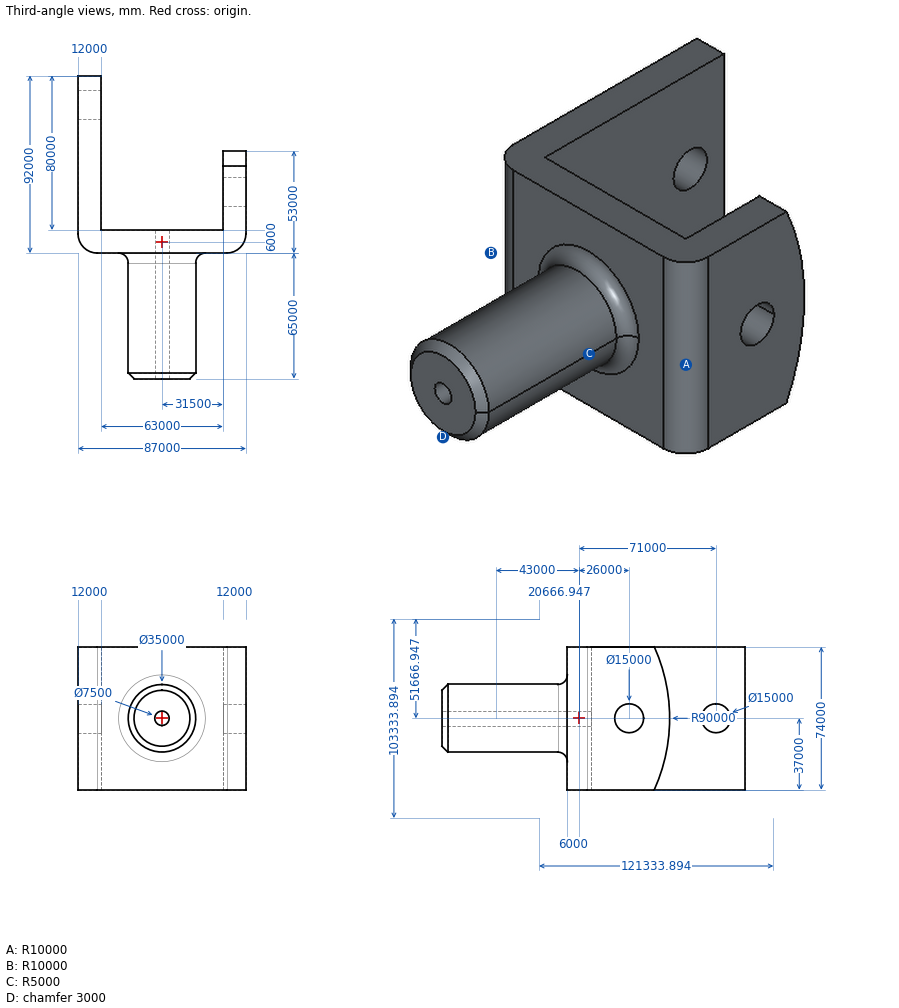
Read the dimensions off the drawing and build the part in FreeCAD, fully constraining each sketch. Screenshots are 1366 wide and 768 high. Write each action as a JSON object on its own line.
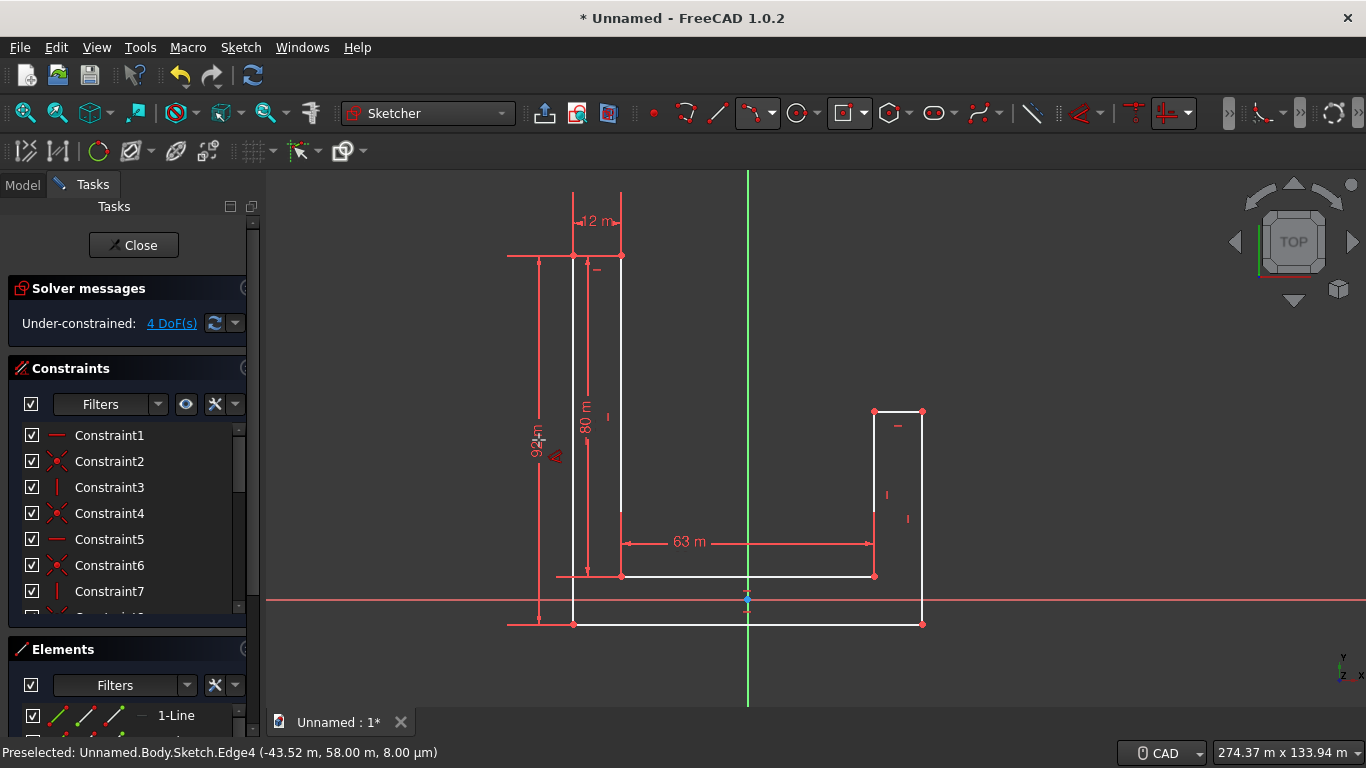
{"action": "left_click", "coordinate": [678, 625]}
{"action": "left_click", "coordinate": [667, 659]}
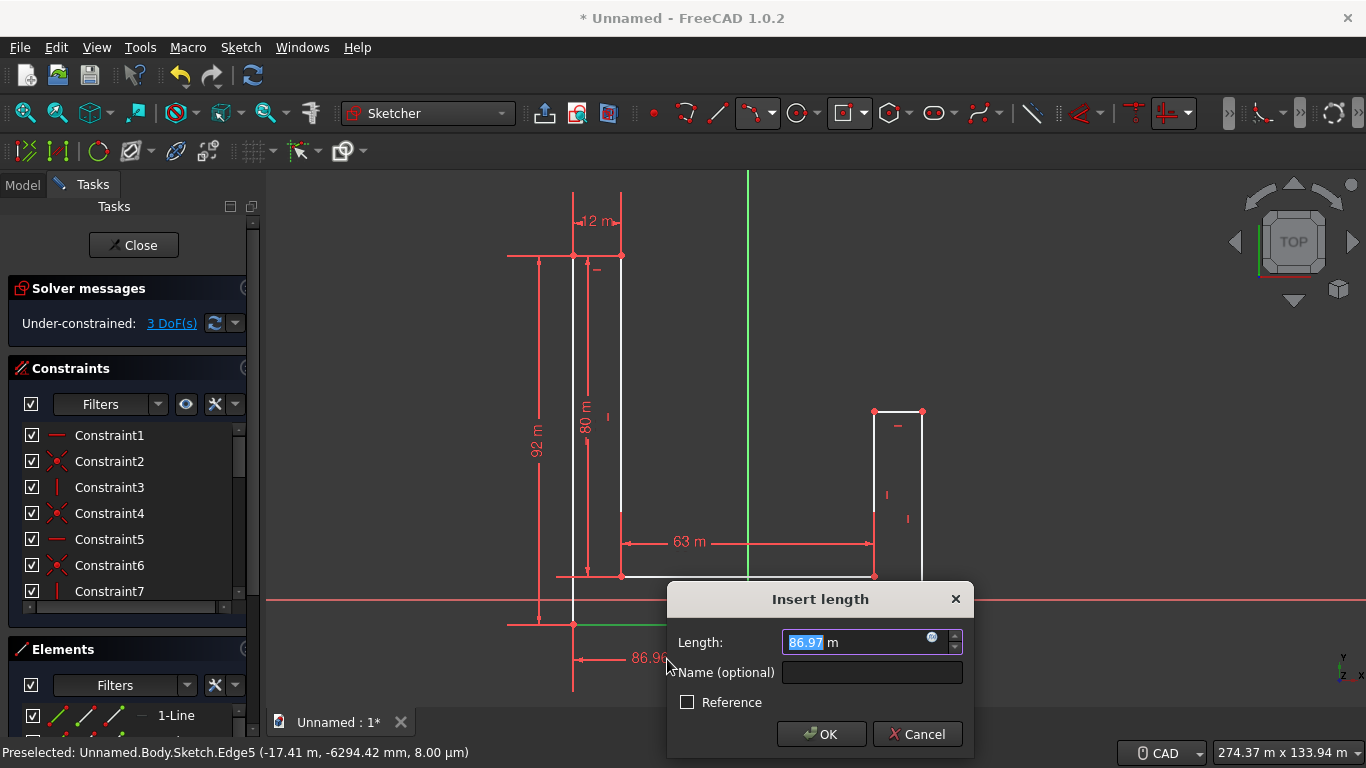
{"action": "key", "text": "ctrl+a"}
{"action": "type", "text": "87000 mm"}
{"action": "key", "text": "Return"}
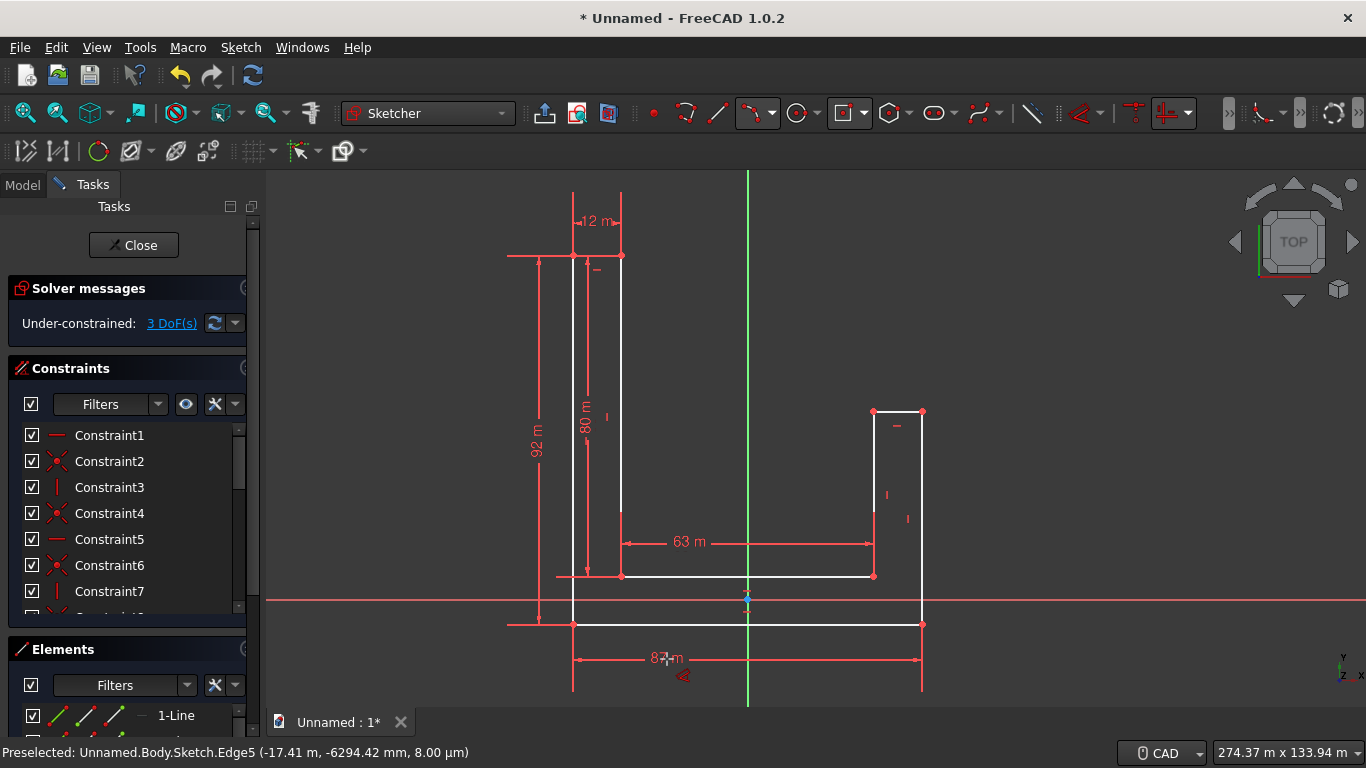
{"action": "left_click", "coordinate": [922, 561]}
{"action": "left_click", "coordinate": [956, 518]}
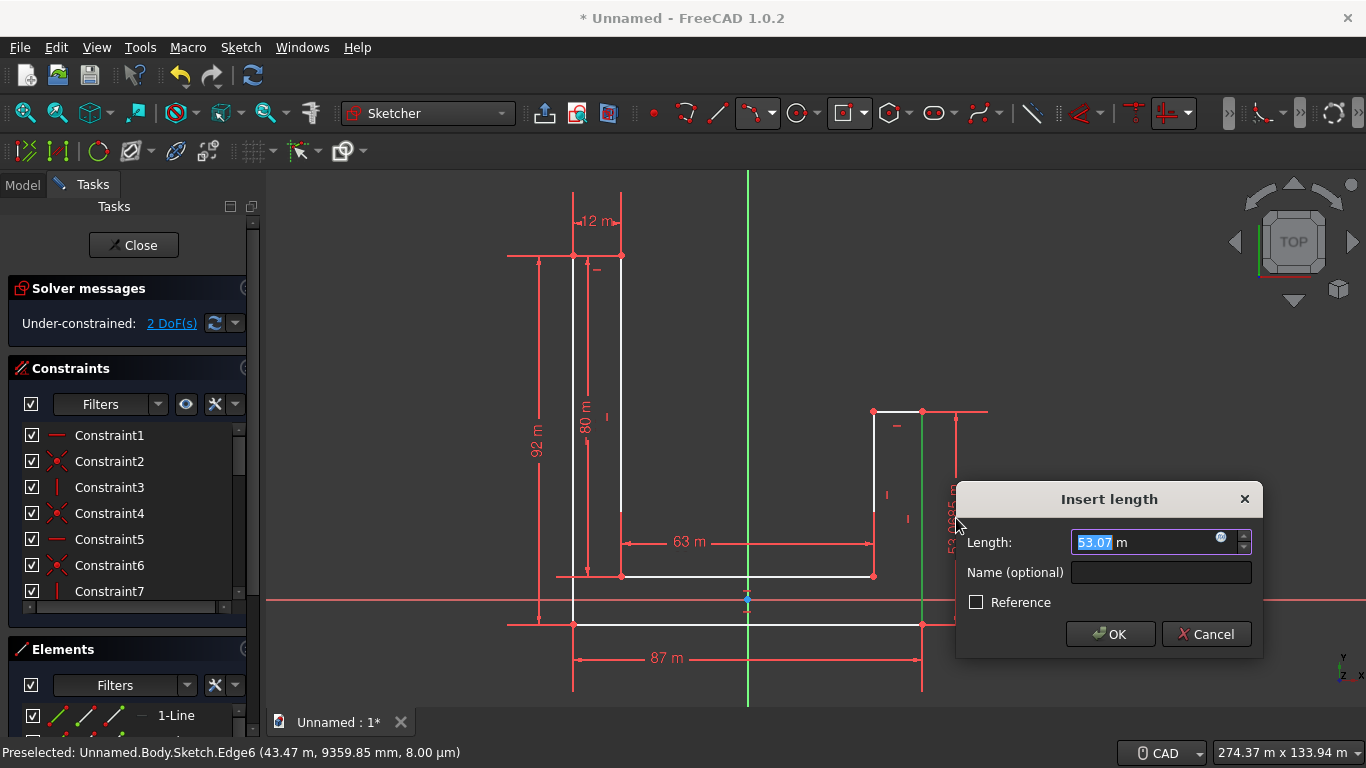
{"action": "key", "text": "ctrl+a"}
{"action": "type", "text": "53000 mm"}
{"action": "key", "text": "Return"}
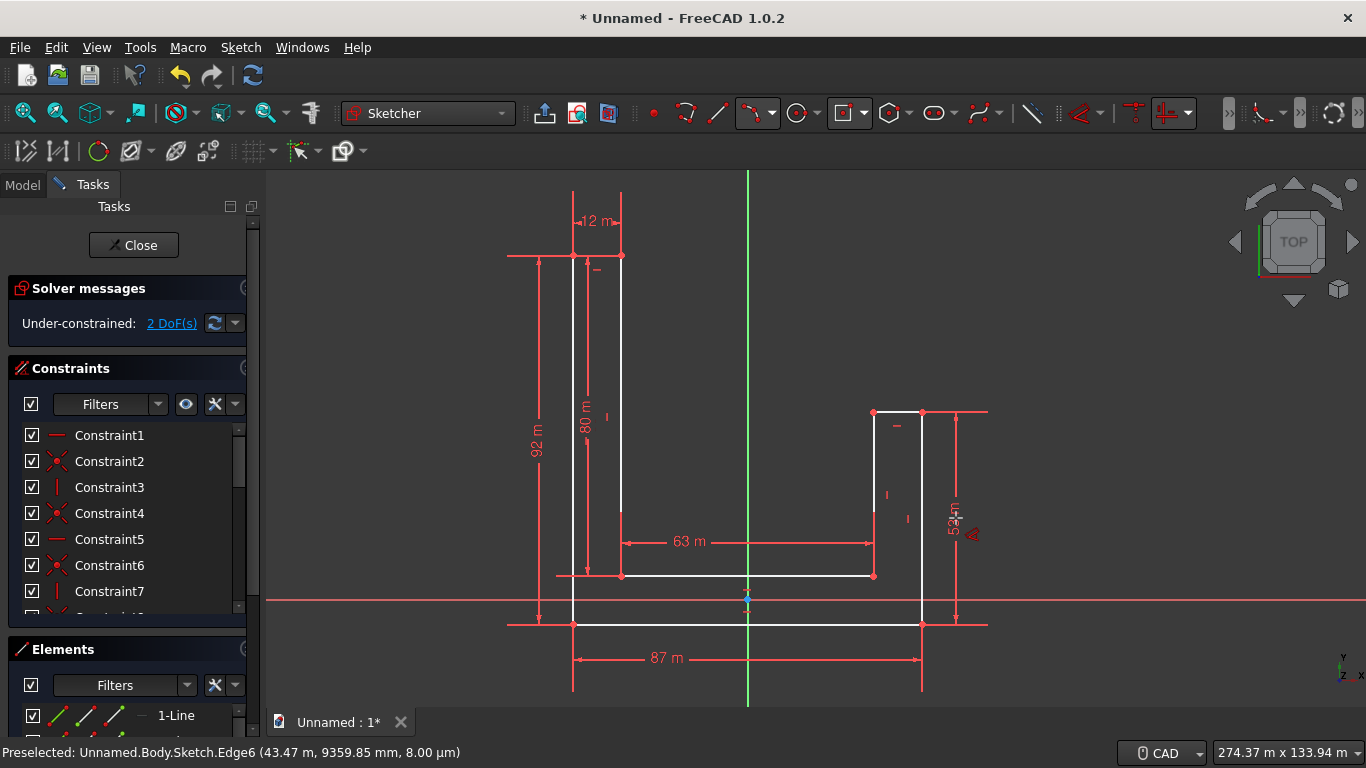
{"action": "scroll", "coordinate": [874, 576], "scroll_direction": "up", "scroll_amount": 3}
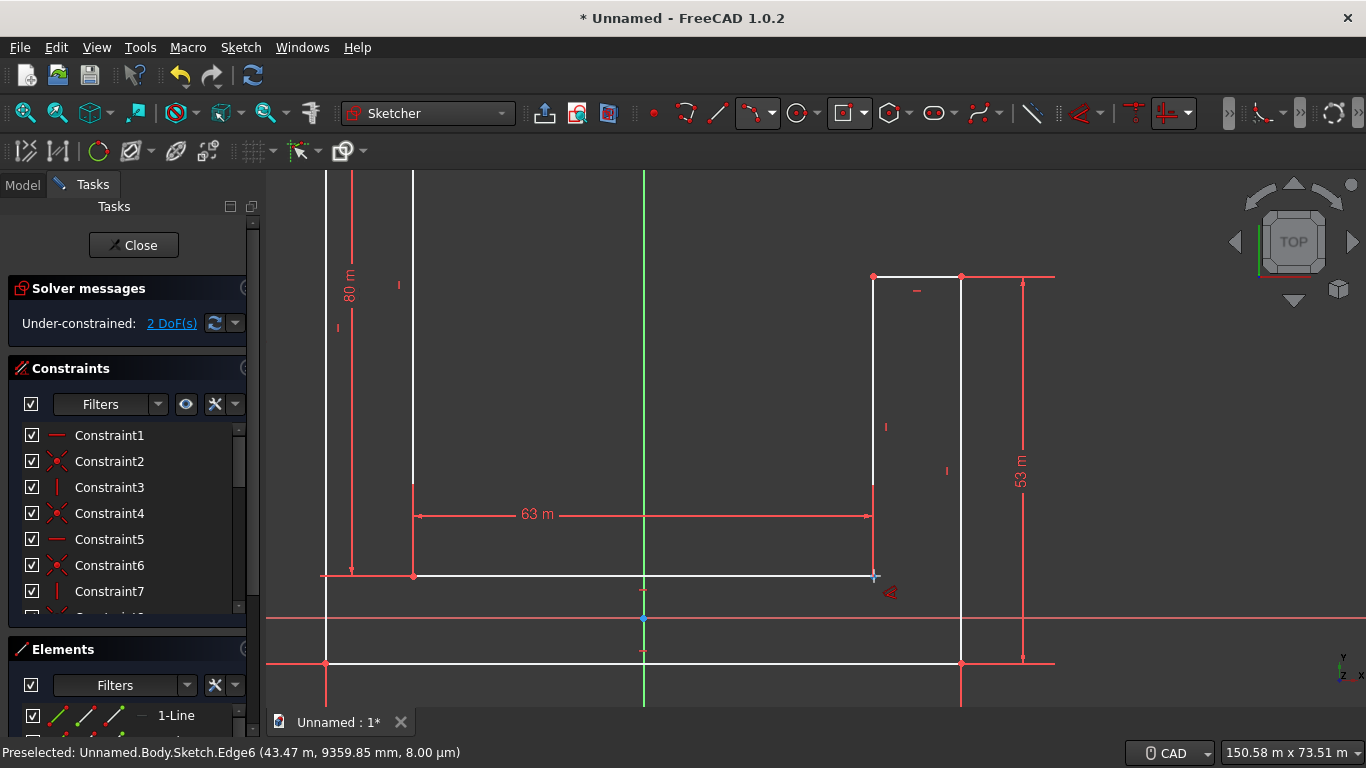
{"action": "left_click", "coordinate": [873, 576]}
{"action": "left_click", "coordinate": [907, 597]}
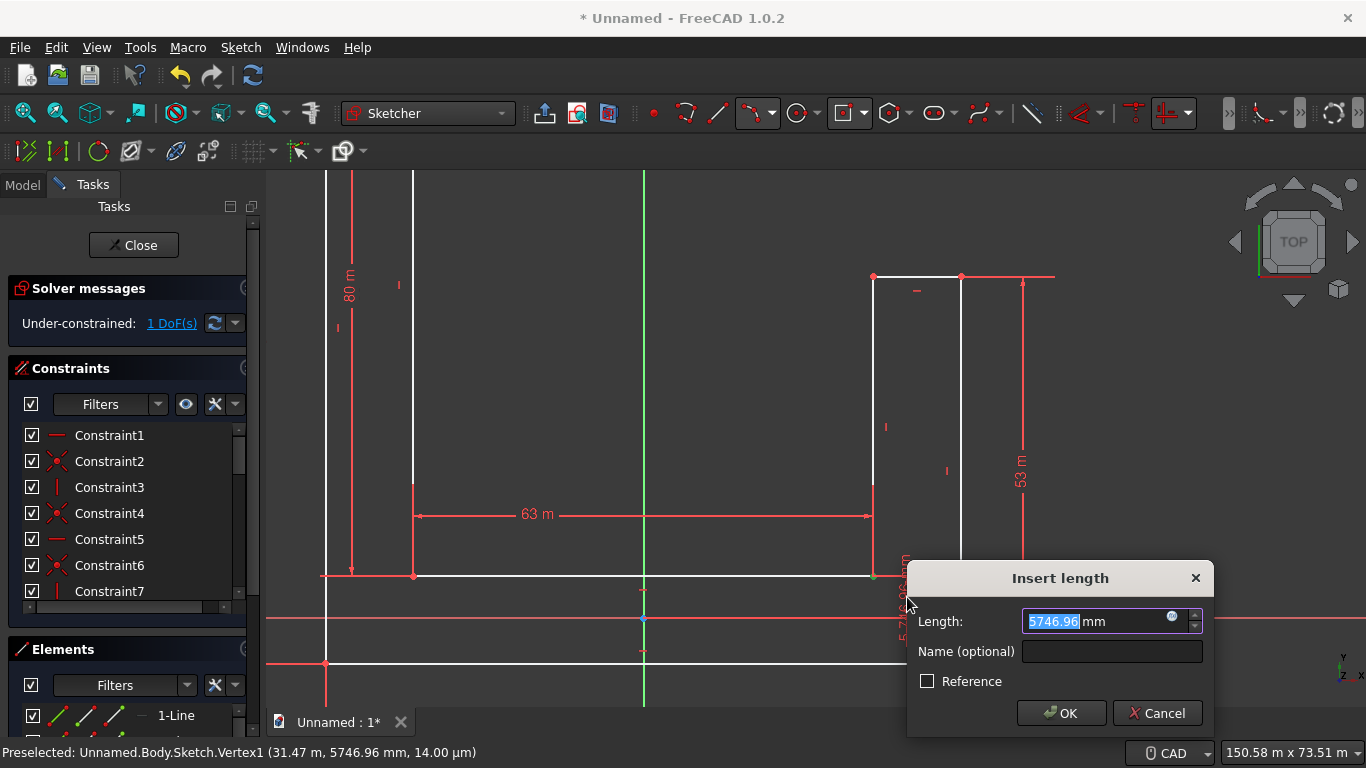
{"action": "type", "text": "6000"}
{"action": "key", "text": "Return"}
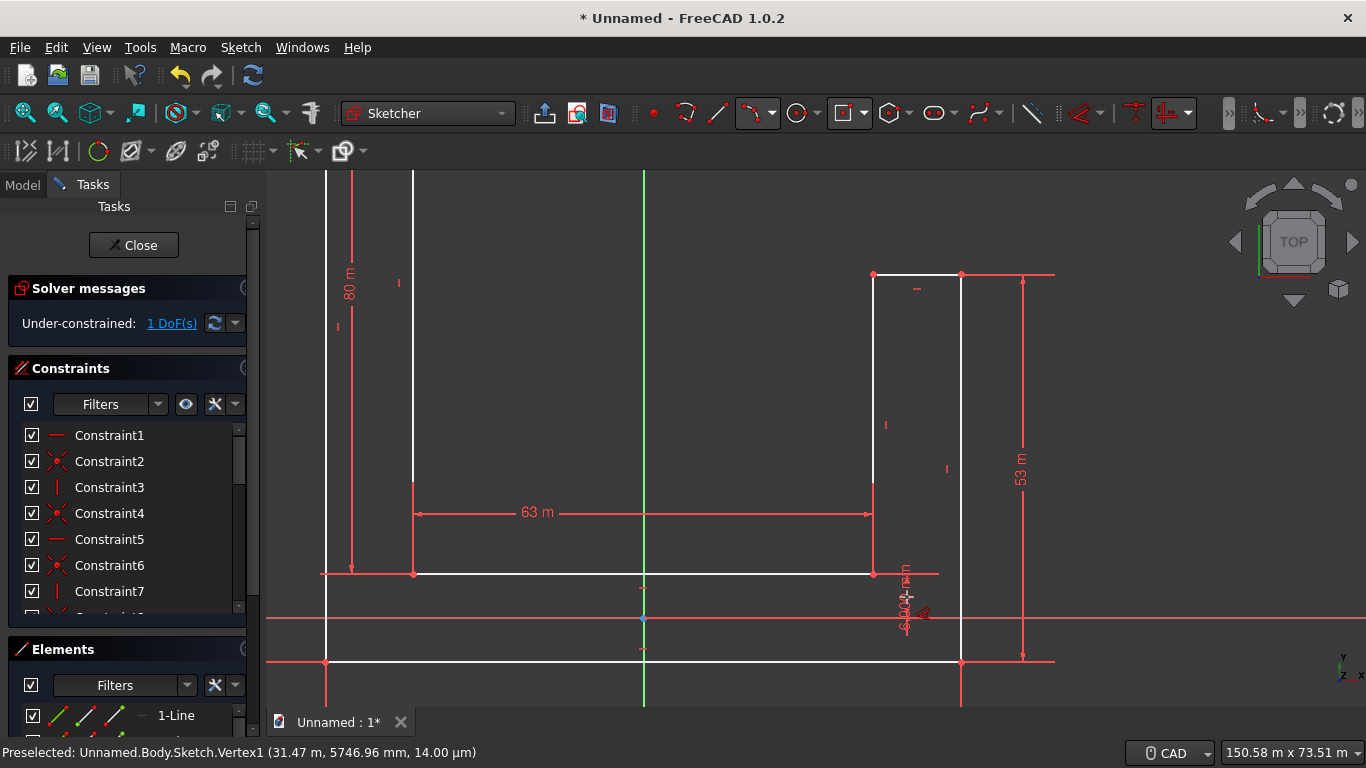
{"action": "left_click", "coordinate": [873, 574]}
{"action": "left_click", "coordinate": [759, 540]}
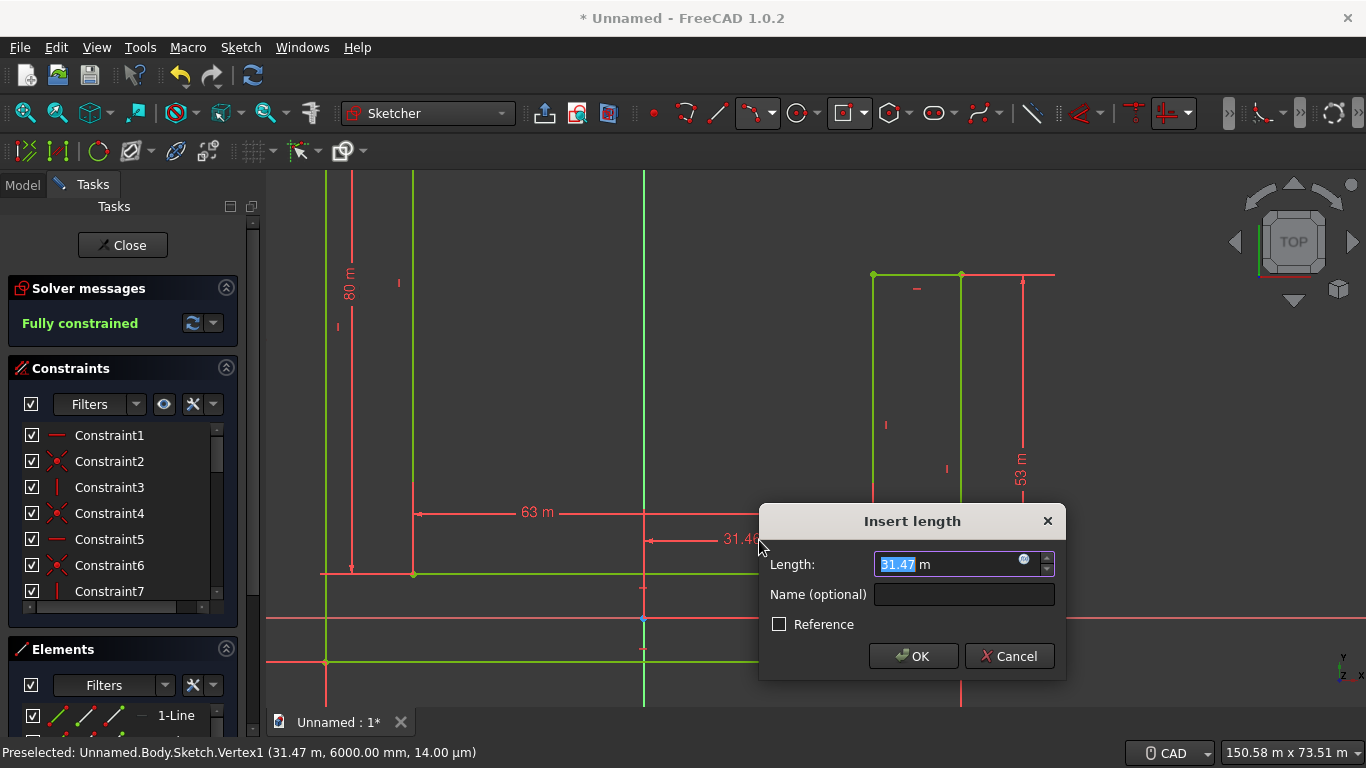
{"action": "key", "text": "ctrl+a"}
{"action": "type", "text": "31500 mm"}
{"action": "key", "text": "Return"}
{"action": "key", "text": "Escape"}